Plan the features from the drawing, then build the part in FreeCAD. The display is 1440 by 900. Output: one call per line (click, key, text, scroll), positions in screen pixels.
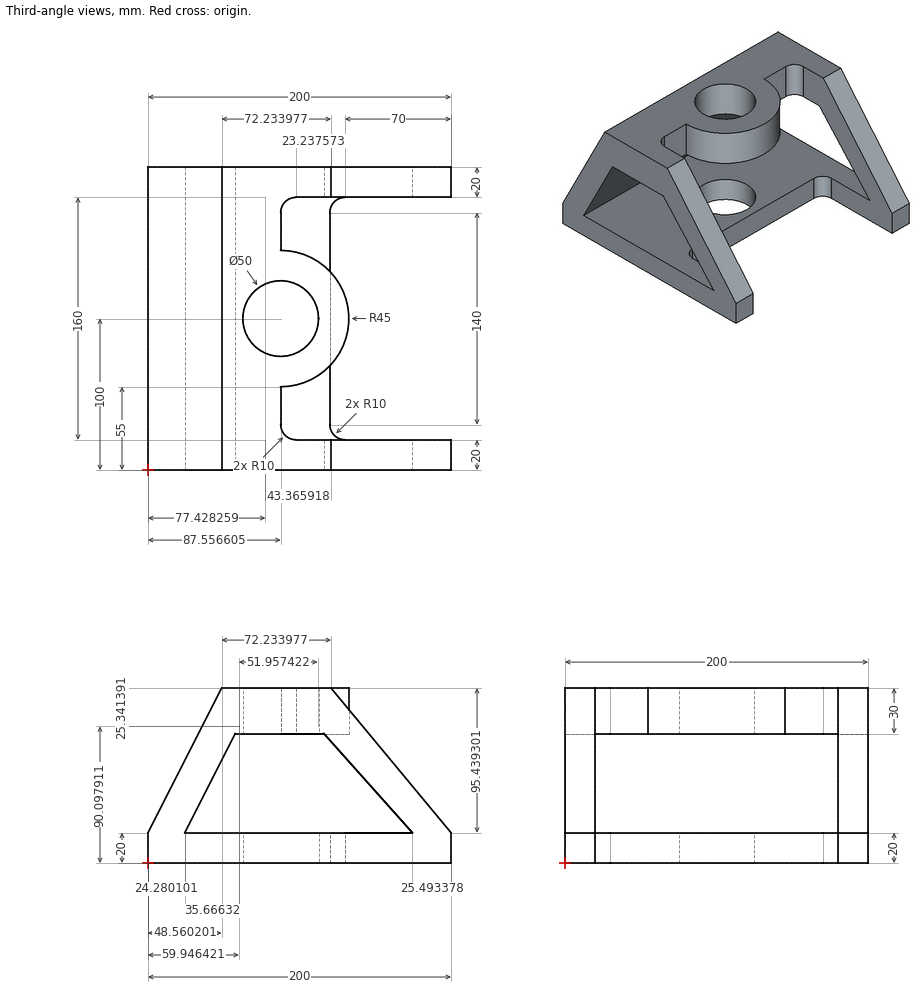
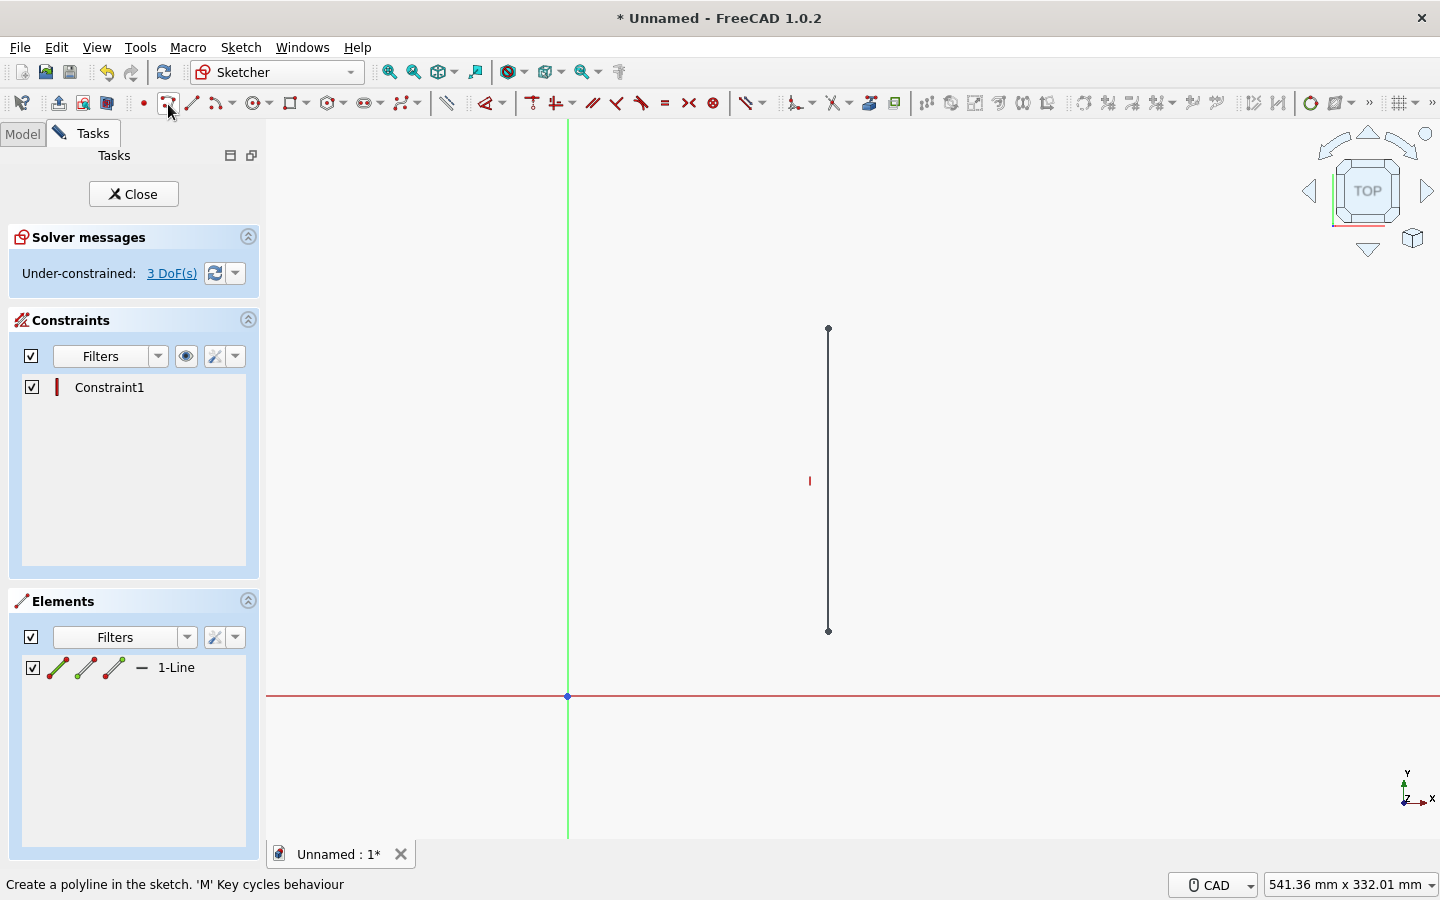
click(850, 306)
click(1002, 306)
click(1002, 263)
click(568, 263)
click(568, 696)
click(1002, 687)
click(1002, 653)
click(850, 653)
right_click(850, 653)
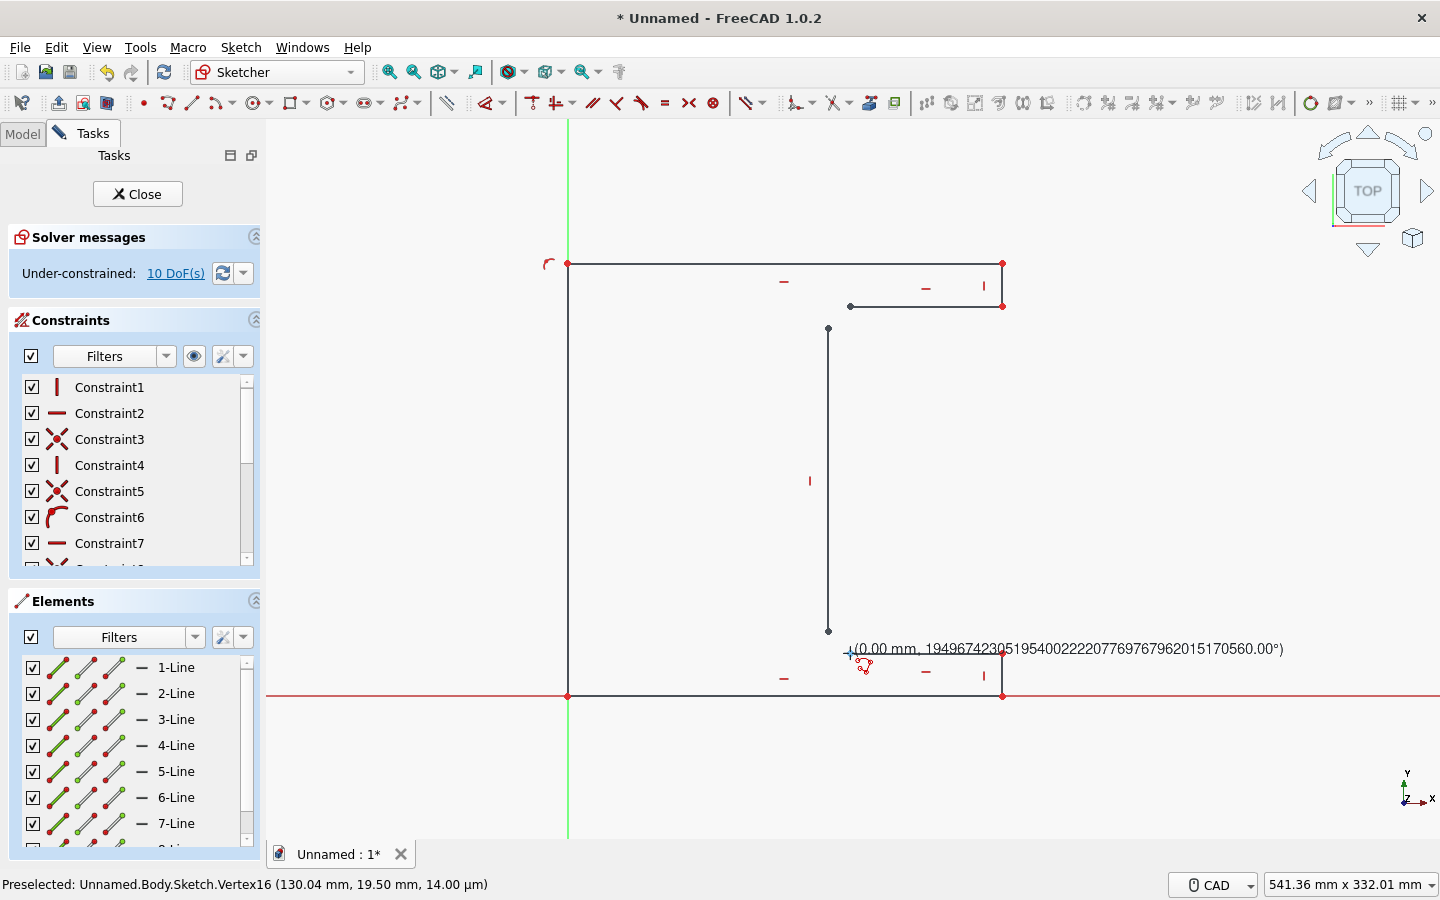
key(g)
key(3)
key(a)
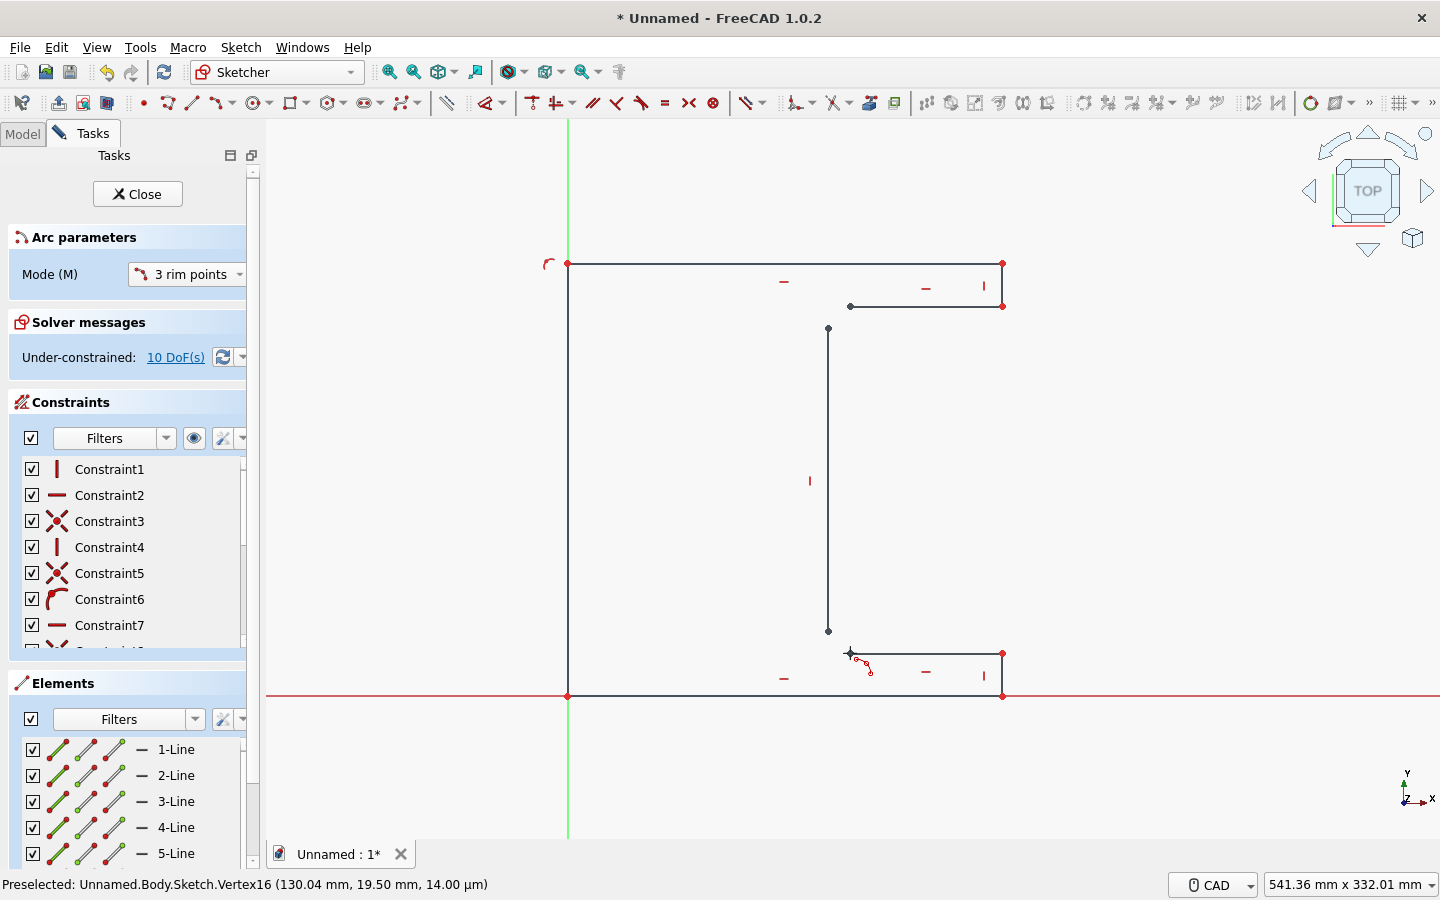
click(828, 329)
click(850, 307)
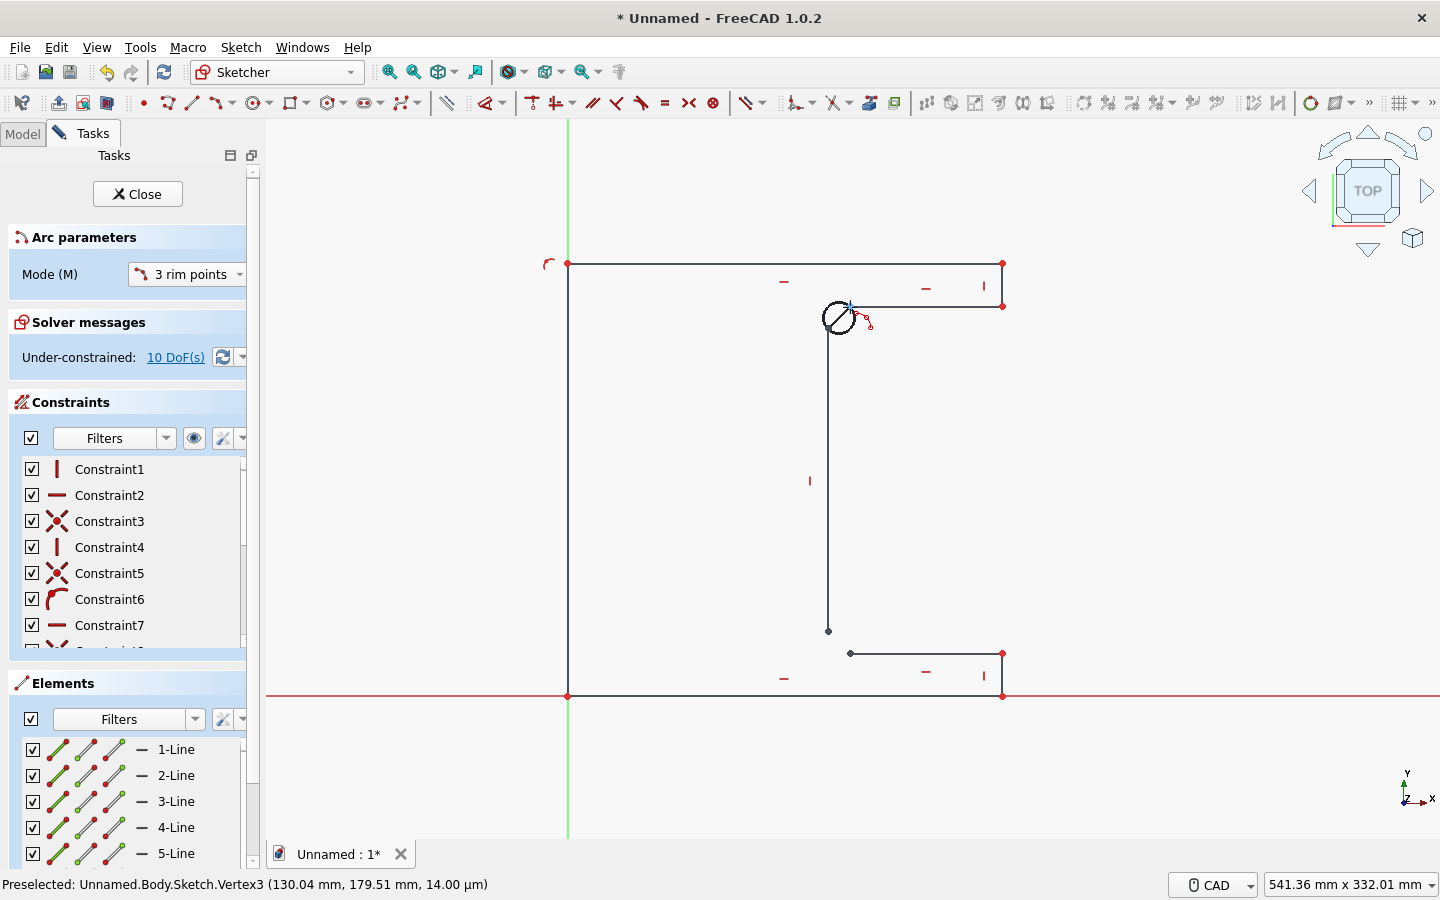
scroll(835, 312, up, 5)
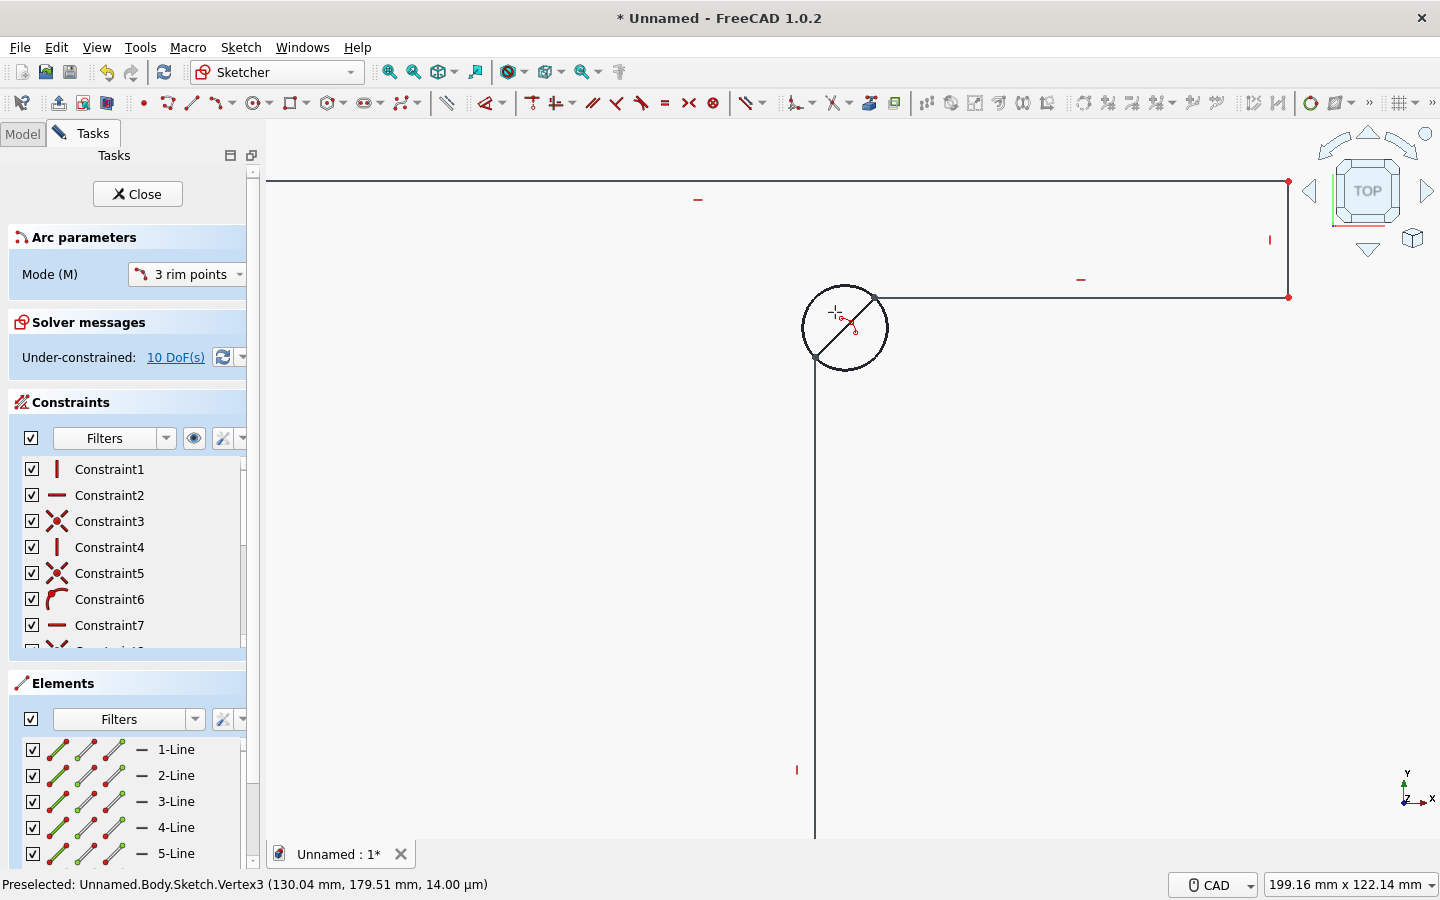
click(833, 312)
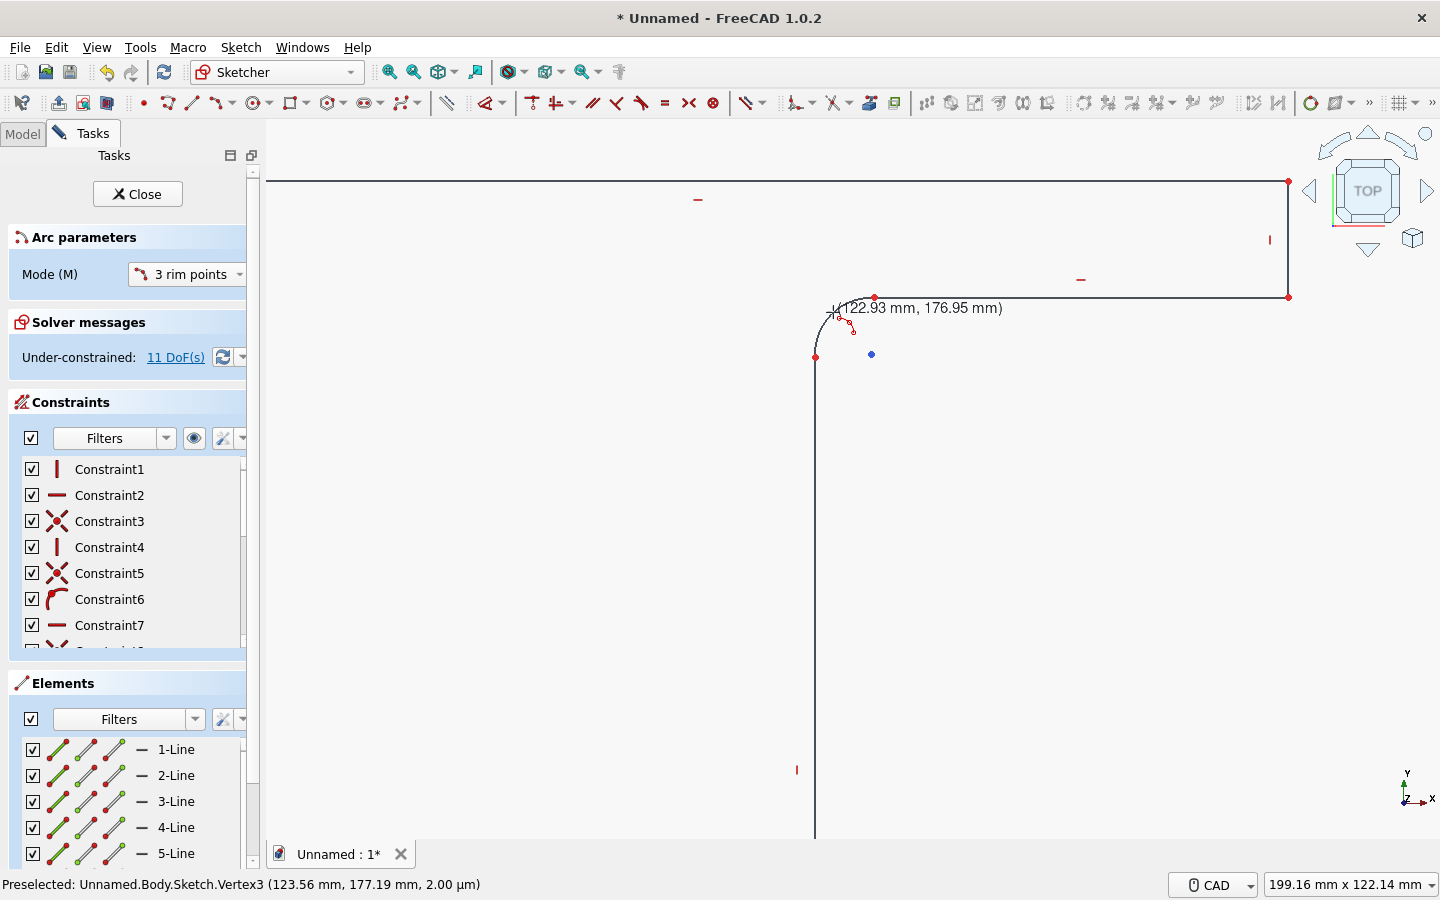
scroll(835, 312, down, 5)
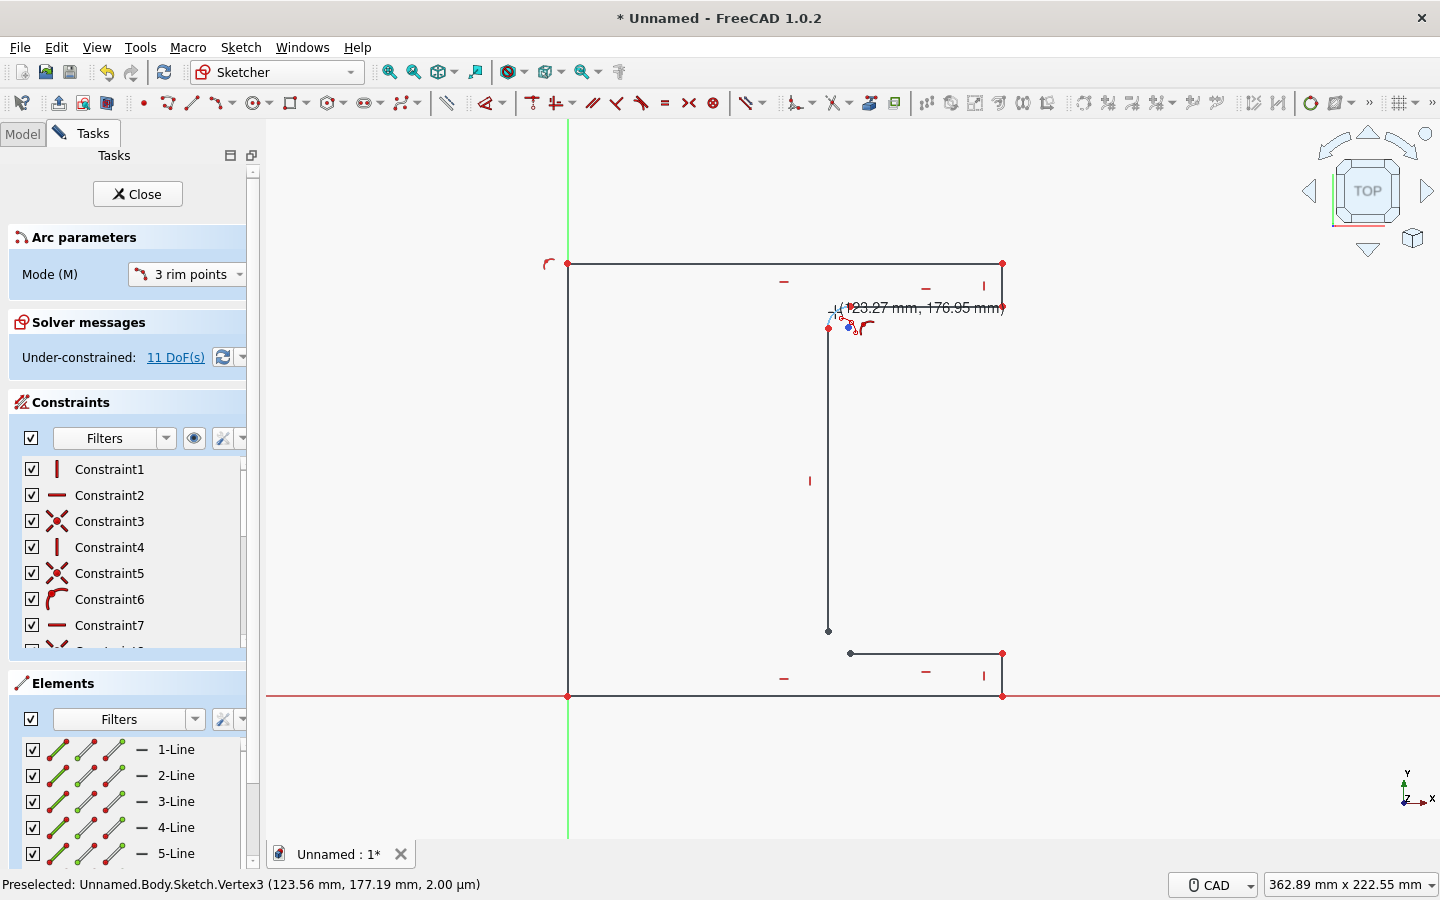
click(850, 654)
click(828, 632)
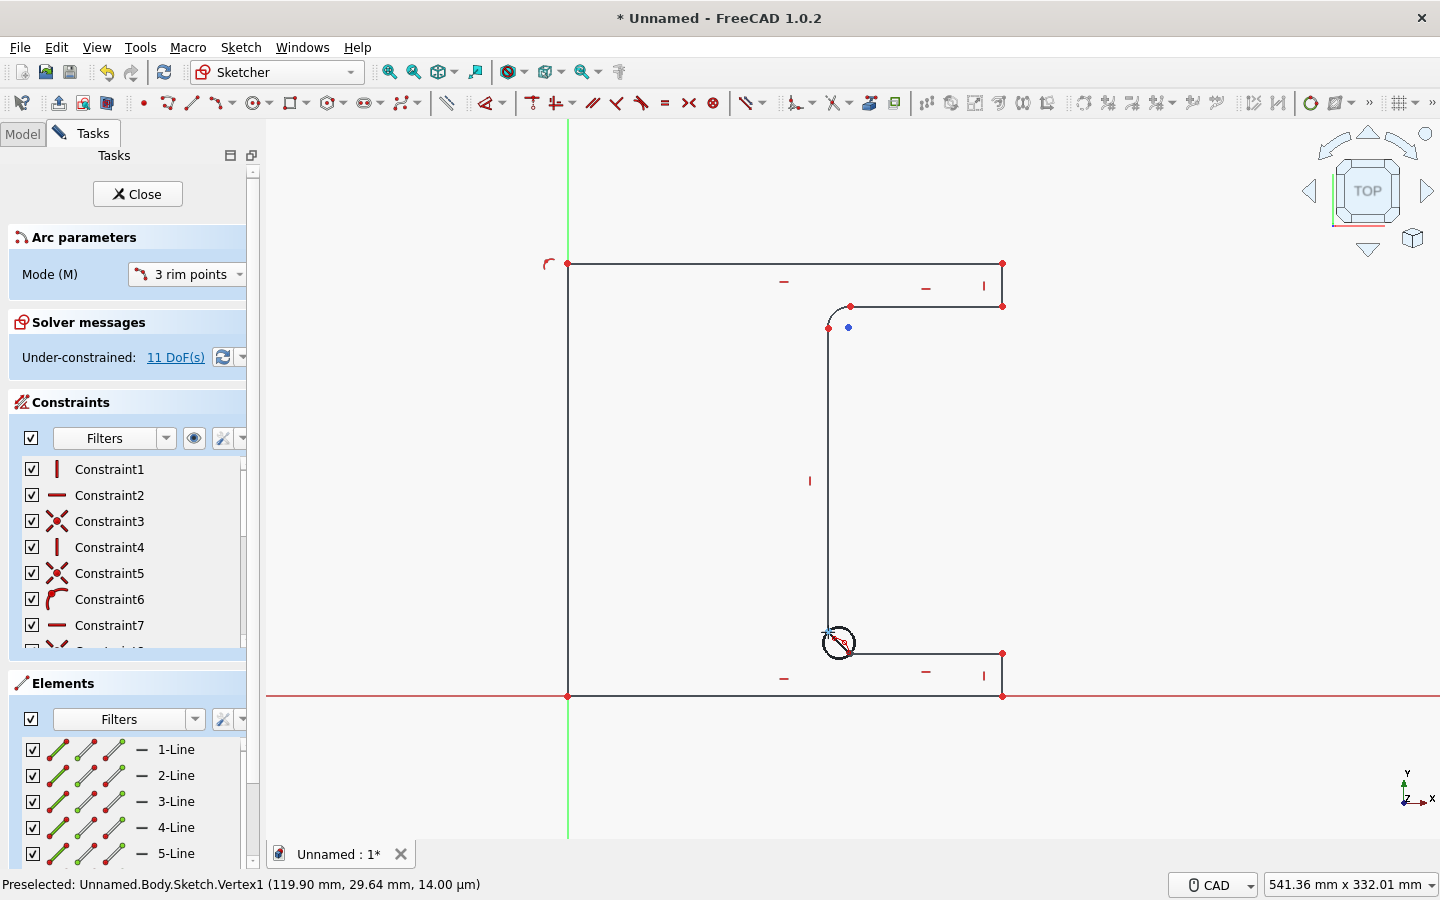
scroll(835, 647, up, 5)